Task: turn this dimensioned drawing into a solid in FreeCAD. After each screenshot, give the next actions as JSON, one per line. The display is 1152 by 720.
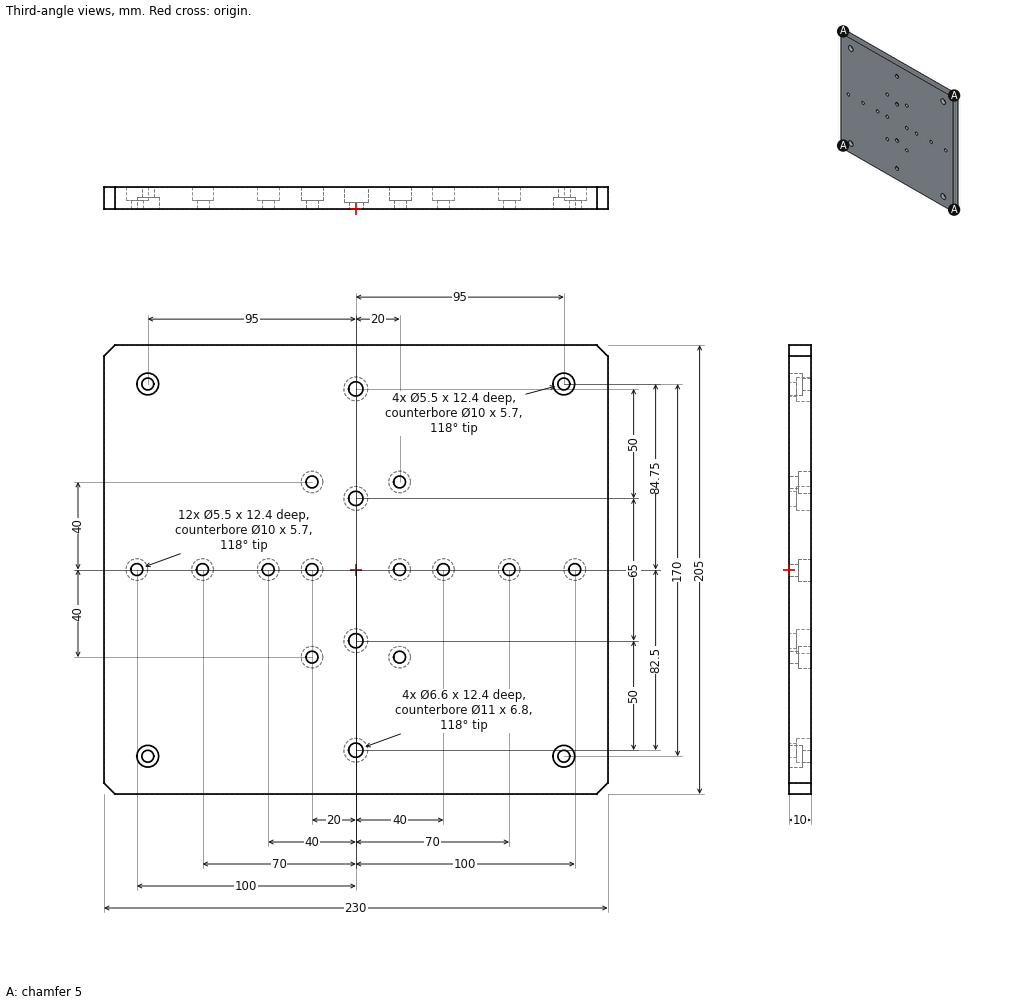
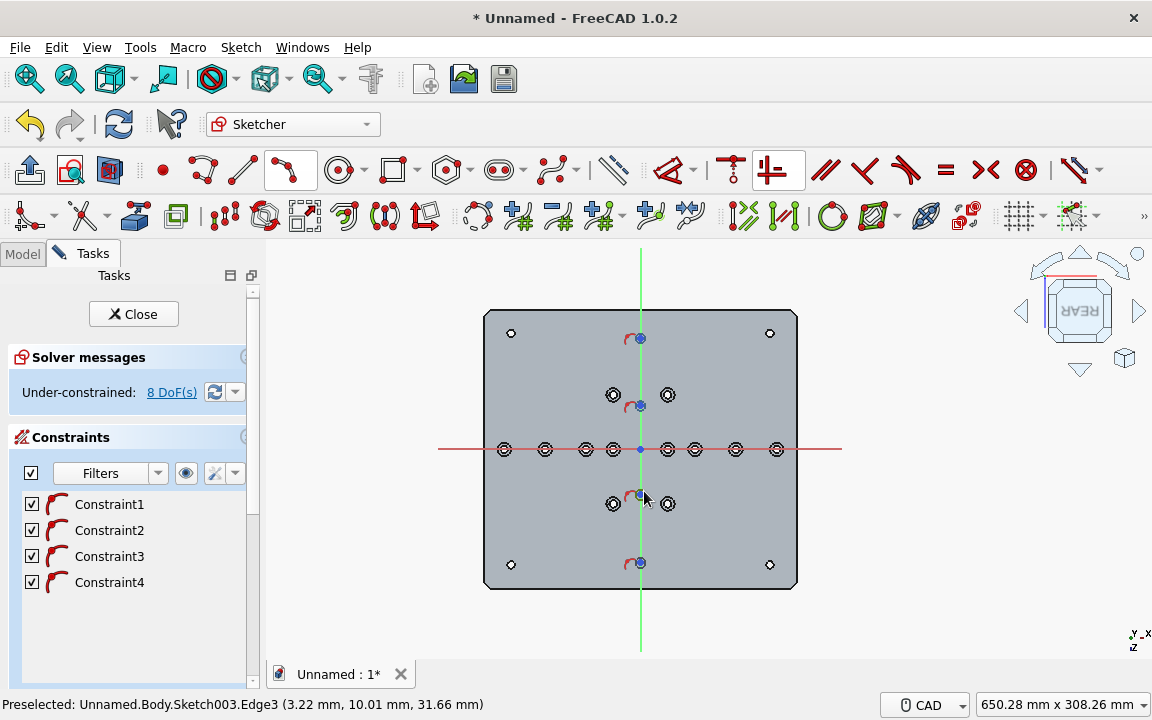
{"action": "scroll", "coordinate": [644, 559], "scroll_direction": "up", "scroll_amount": 7}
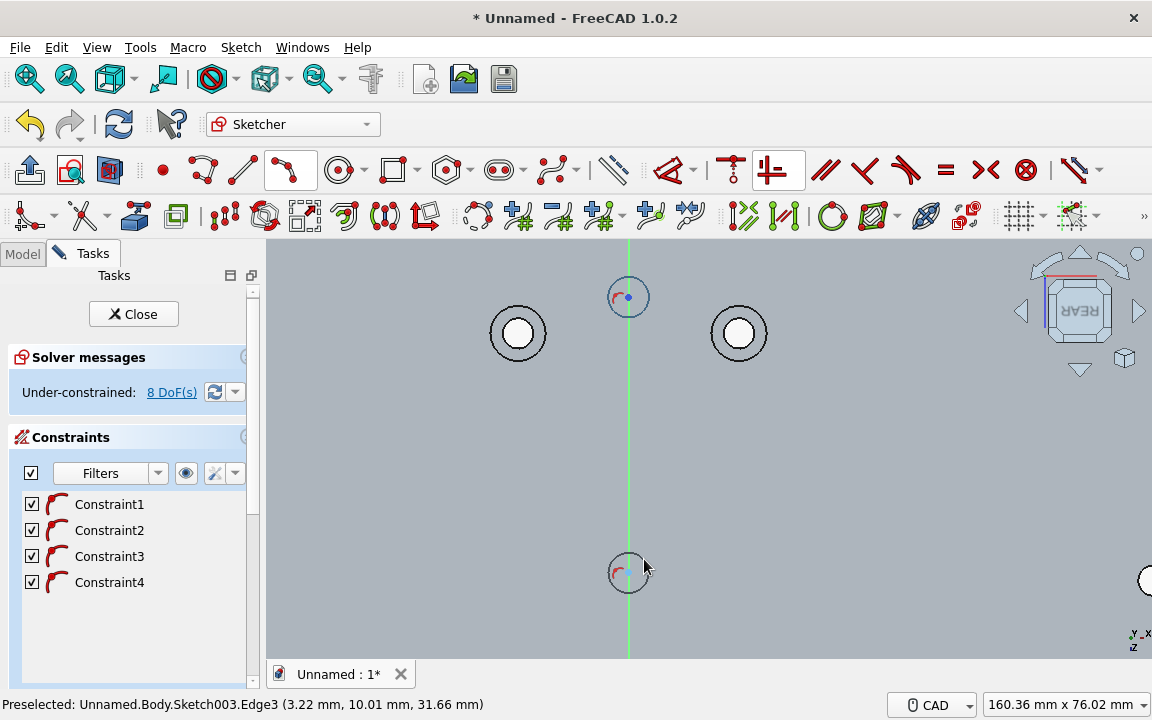
{"action": "left_click", "coordinate": [643, 559]}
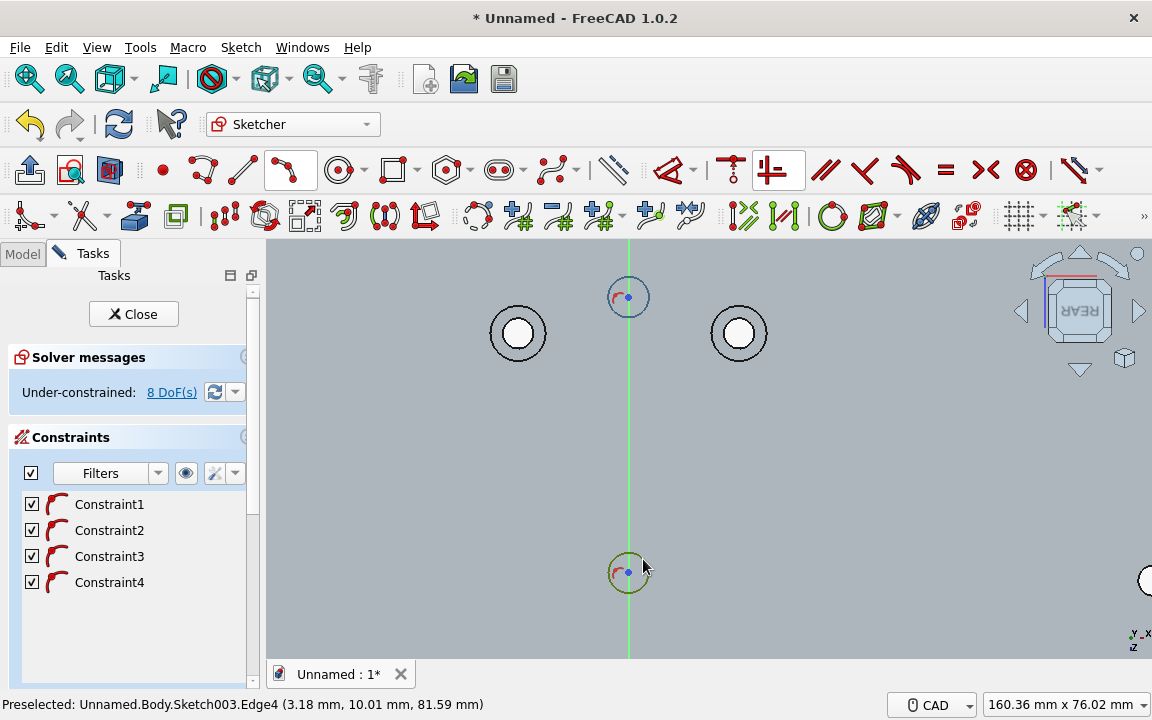
{"action": "left_click", "coordinate": [946, 170]}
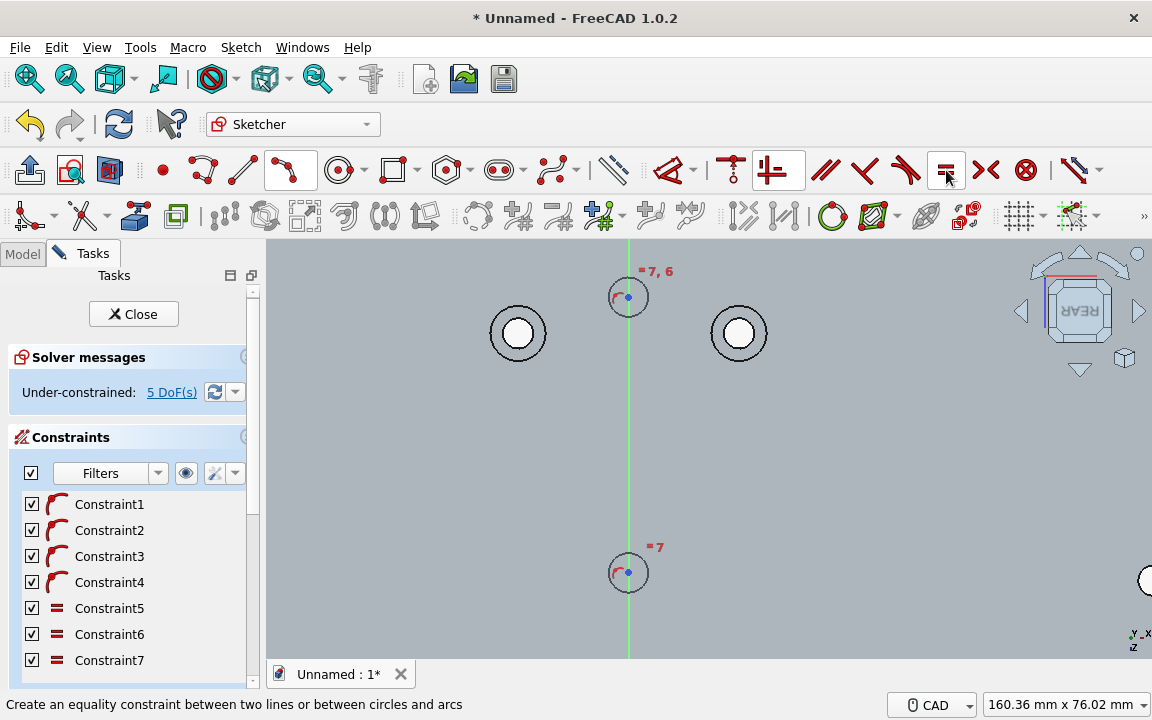
{"action": "left_click", "coordinate": [668, 170]}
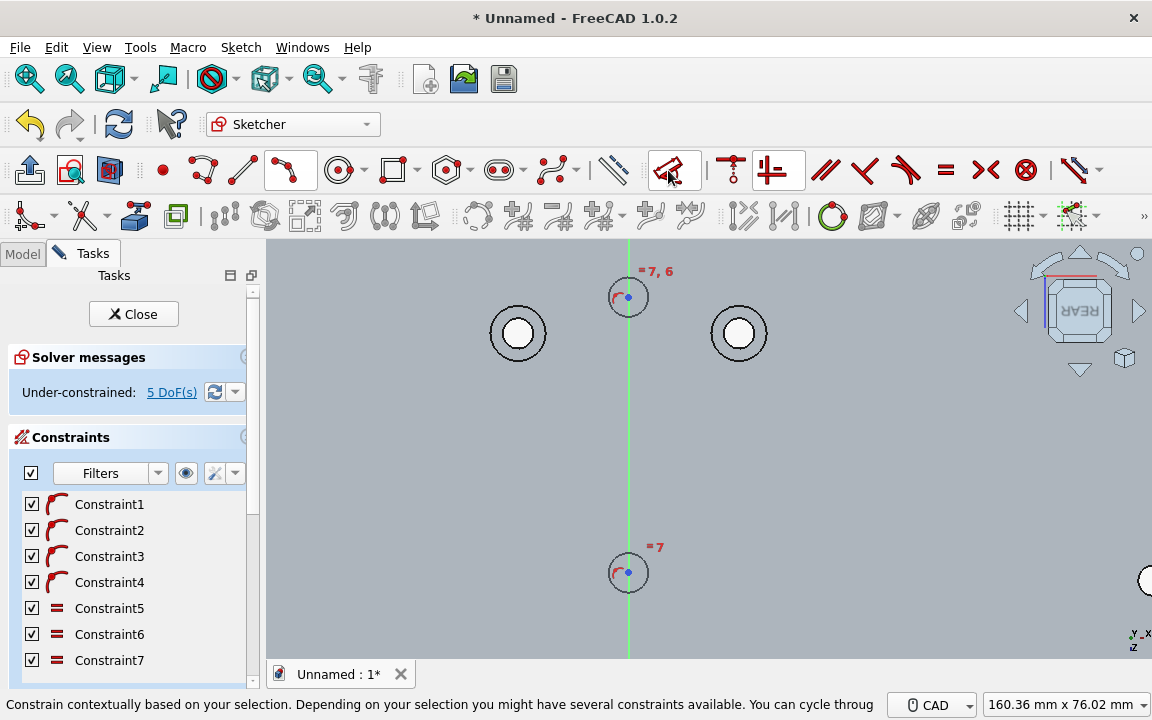
{"action": "scroll", "coordinate": [644, 559], "scroll_direction": "down", "scroll_amount": 7}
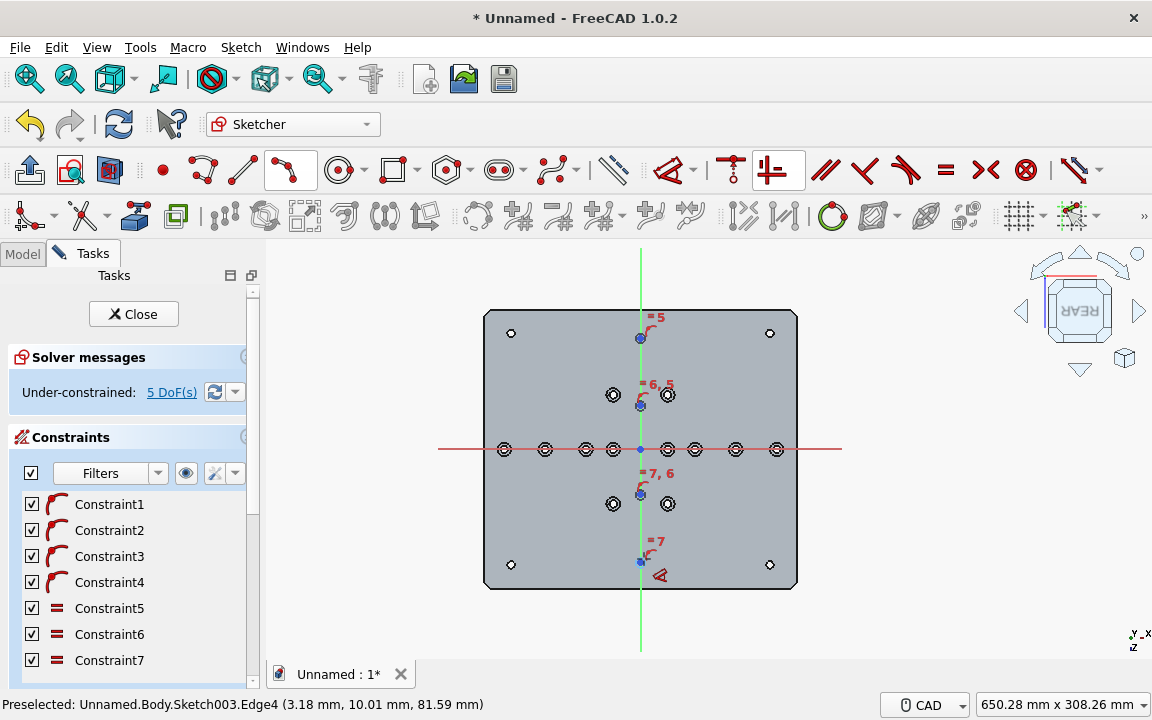
{"action": "scroll", "coordinate": [644, 335], "scroll_direction": "up", "scroll_amount": 8}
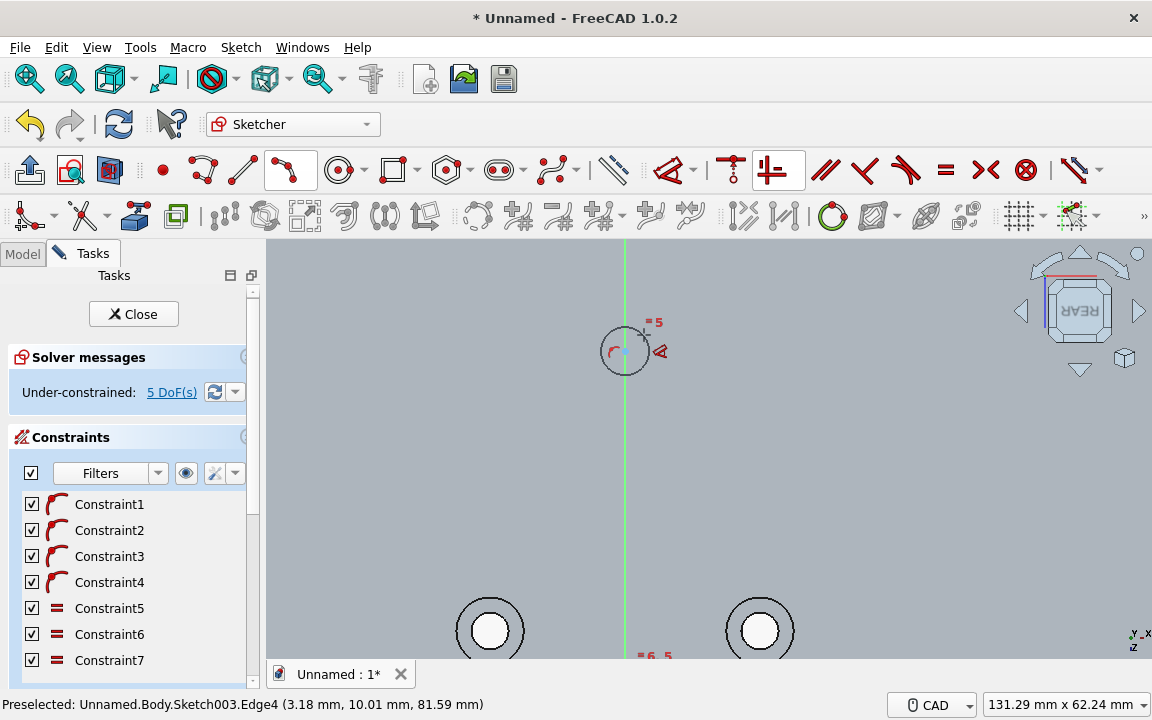
{"action": "left_click", "coordinate": [642, 334]}
{"action": "left_click", "coordinate": [664, 311]}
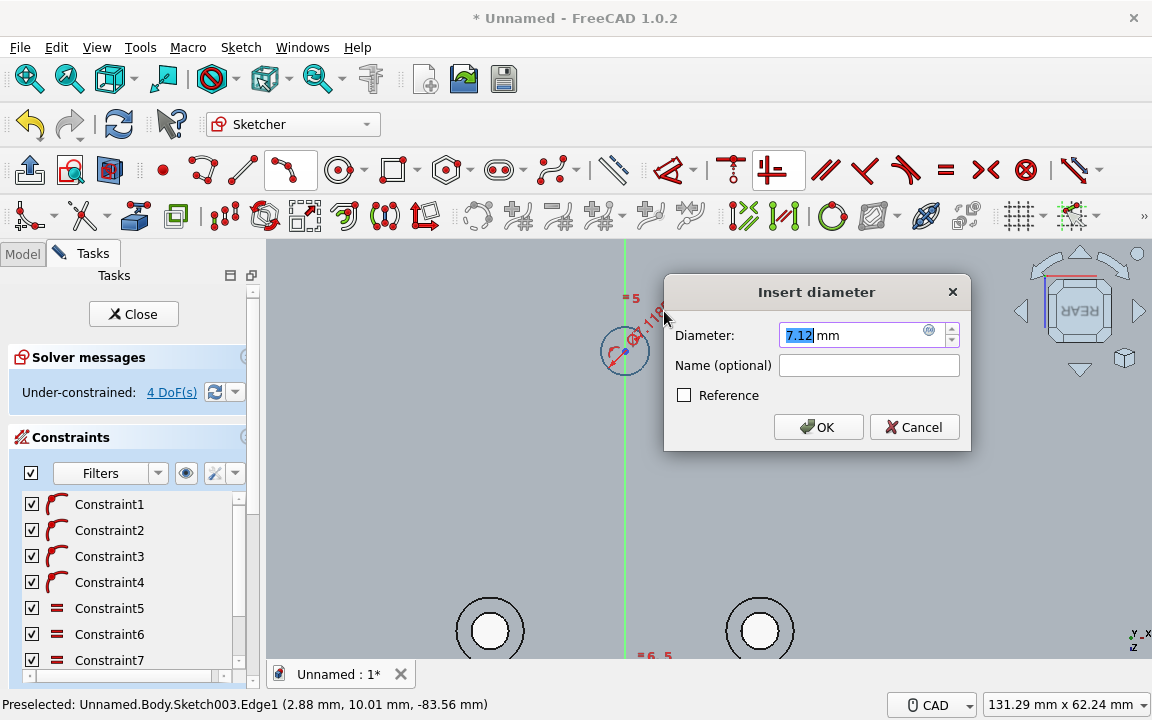
{"action": "type", "text": "6.6"}
{"action": "key", "text": "Return"}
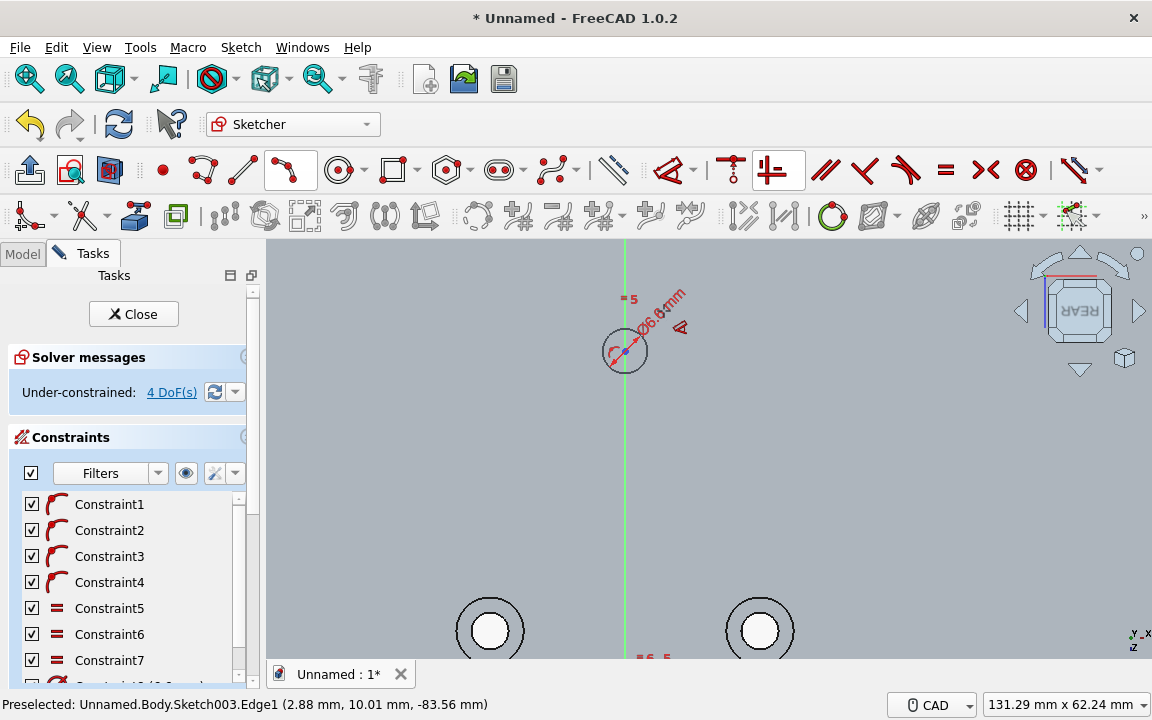
{"action": "scroll", "coordinate": [644, 335], "scroll_direction": "down", "scroll_amount": 8}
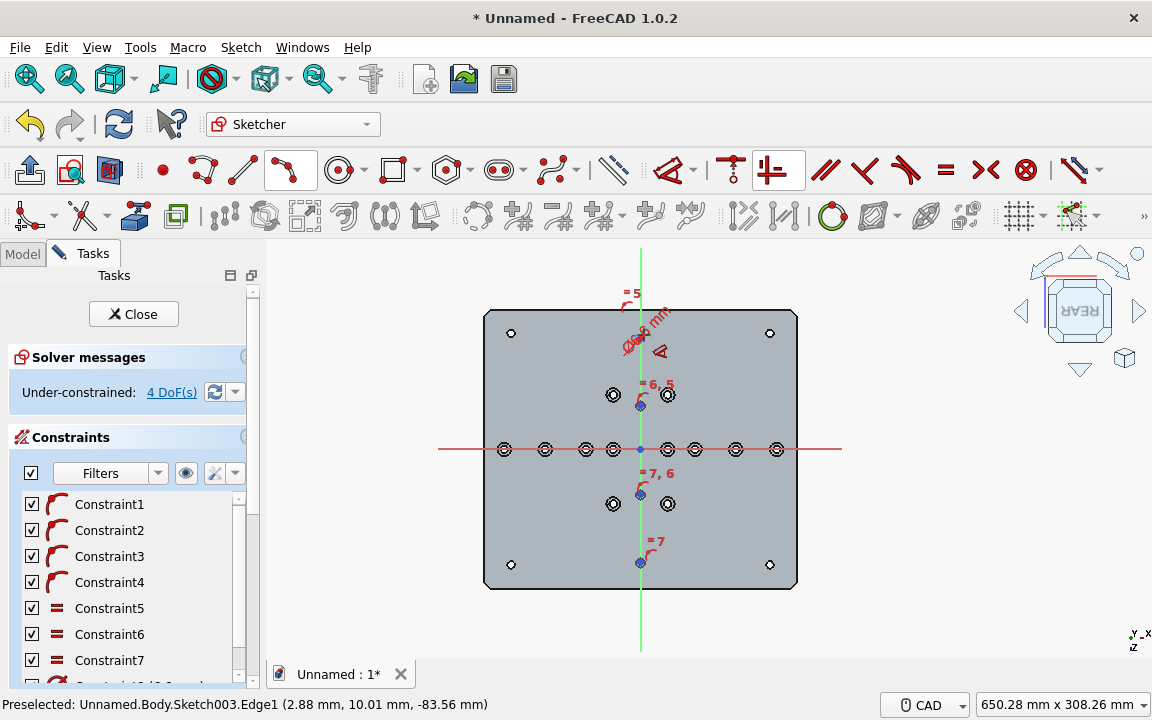
{"action": "left_click", "coordinate": [641, 338]}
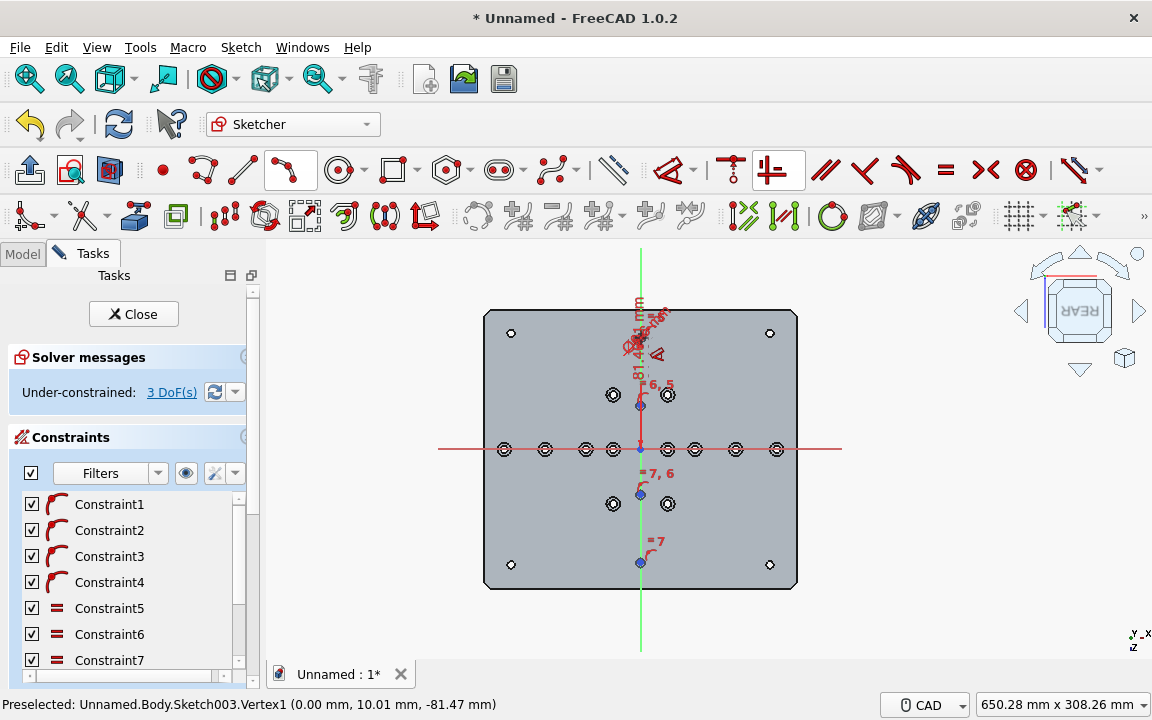
{"action": "left_click", "coordinate": [641, 406]}
{"action": "left_click", "coordinate": [675, 372]}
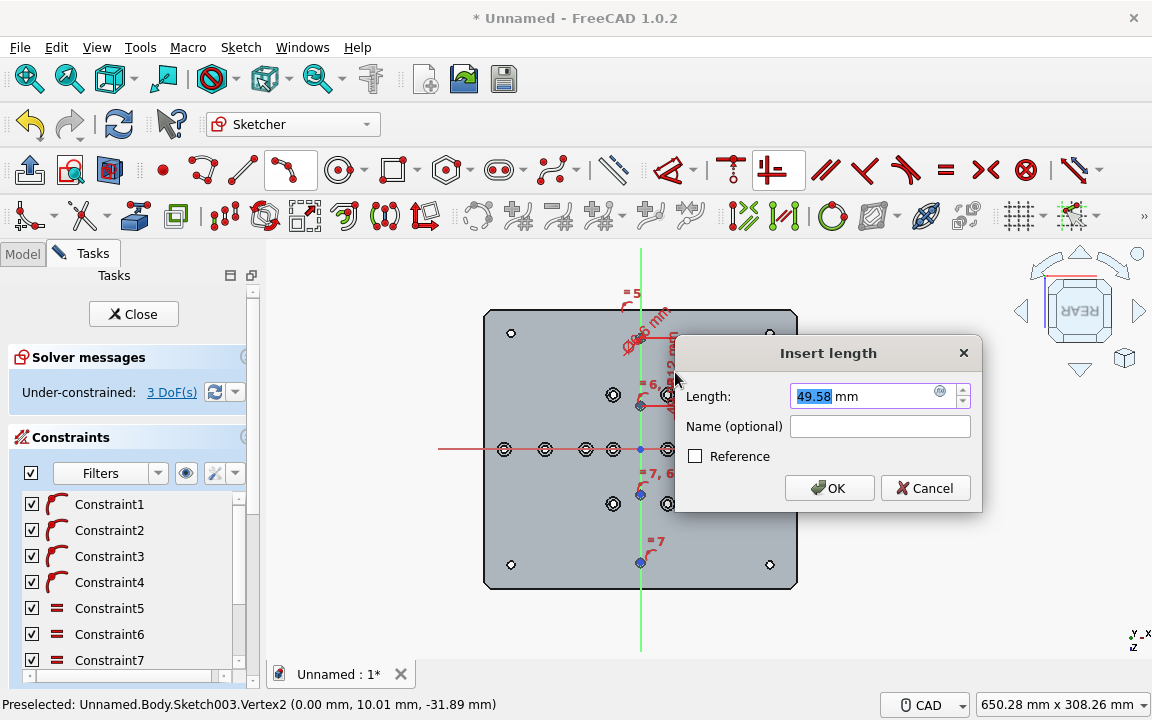
{"action": "type", "text": "50"}
{"action": "key", "text": "Return"}